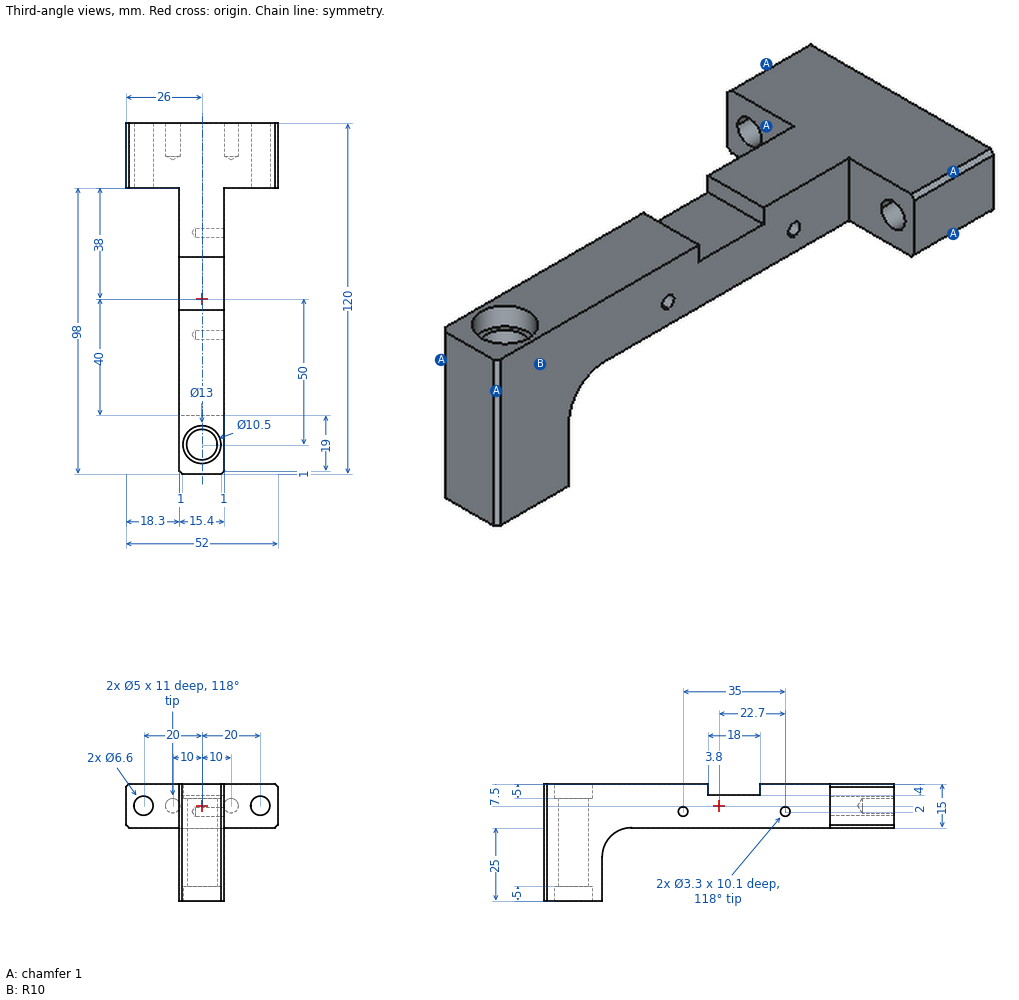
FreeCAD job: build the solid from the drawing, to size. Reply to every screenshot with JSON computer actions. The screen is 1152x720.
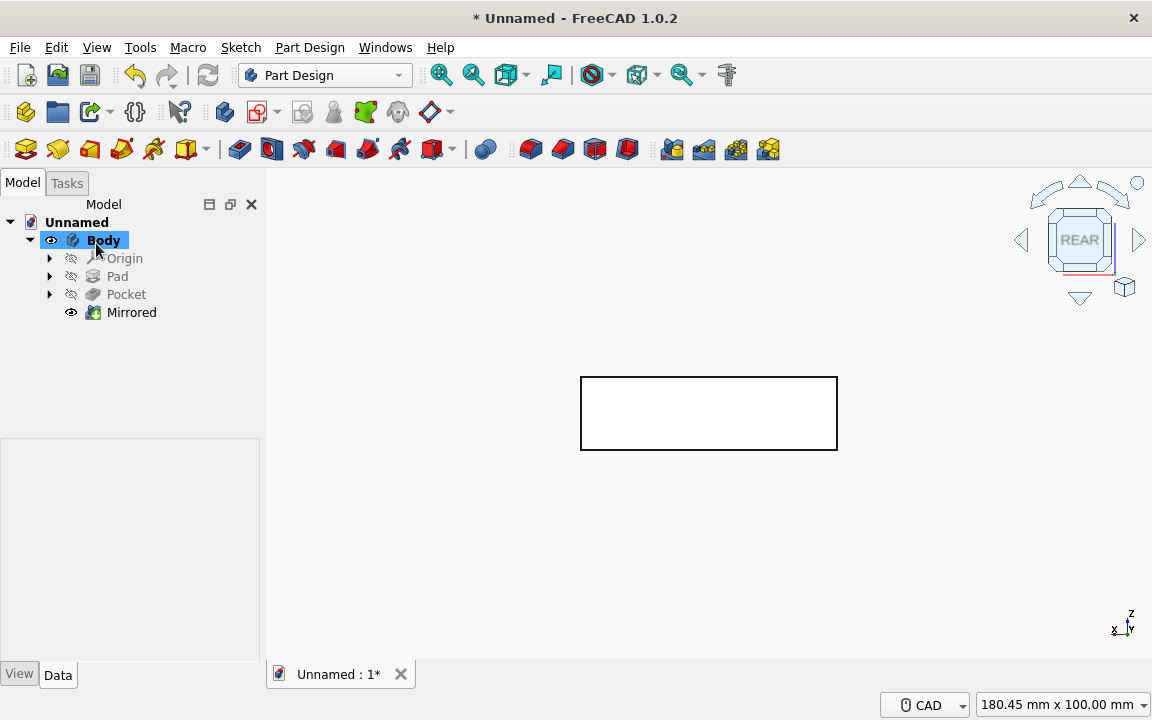
{"action": "left_click", "coordinate": [442, 76]}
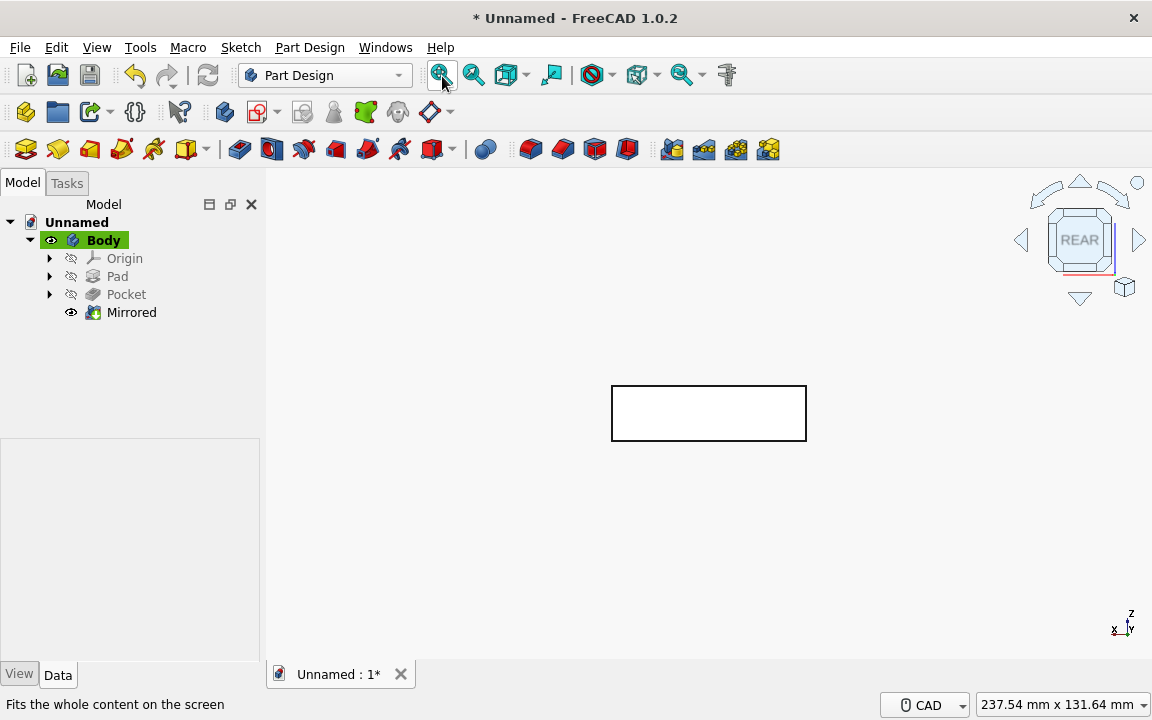
{"action": "left_click", "coordinate": [654, 413]}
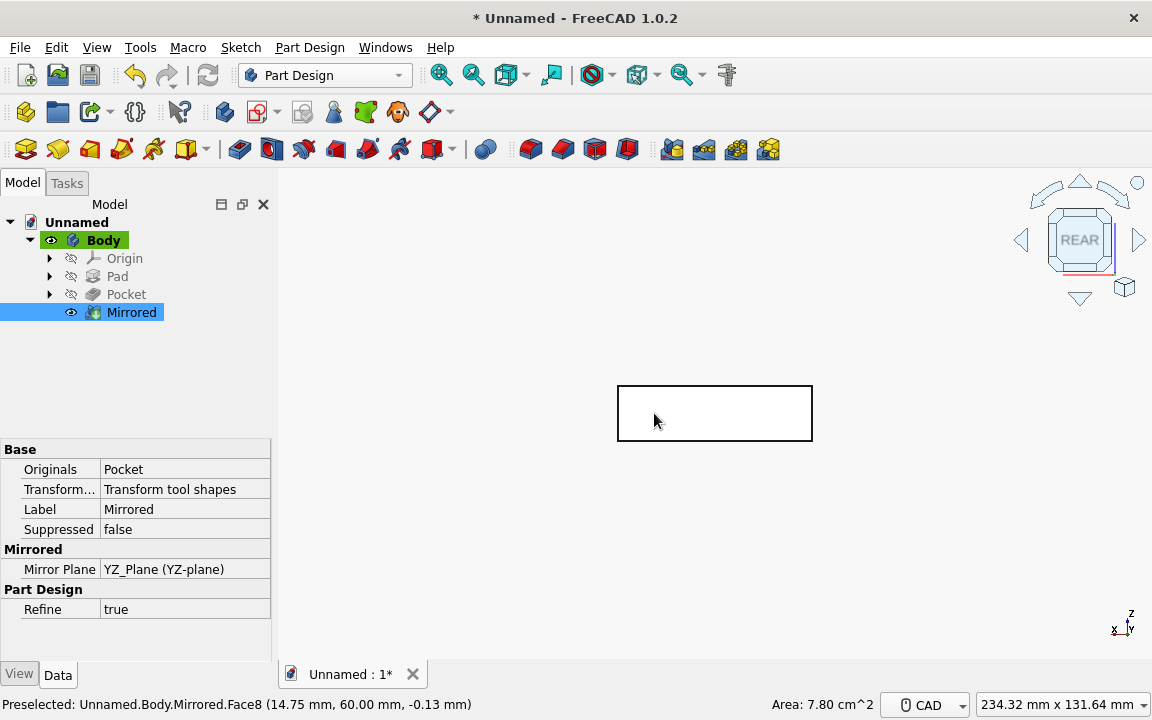
{"action": "left_click", "coordinate": [258, 112]}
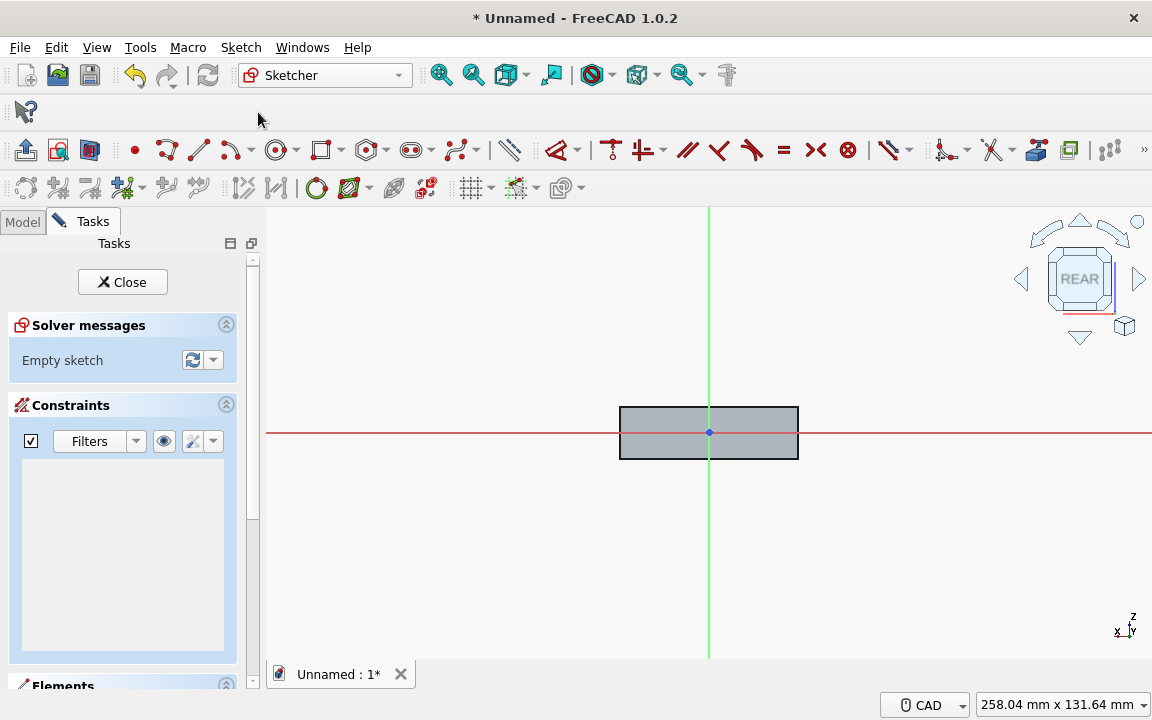
{"action": "scroll", "coordinate": [739, 433], "scroll_direction": "up", "scroll_amount": 6}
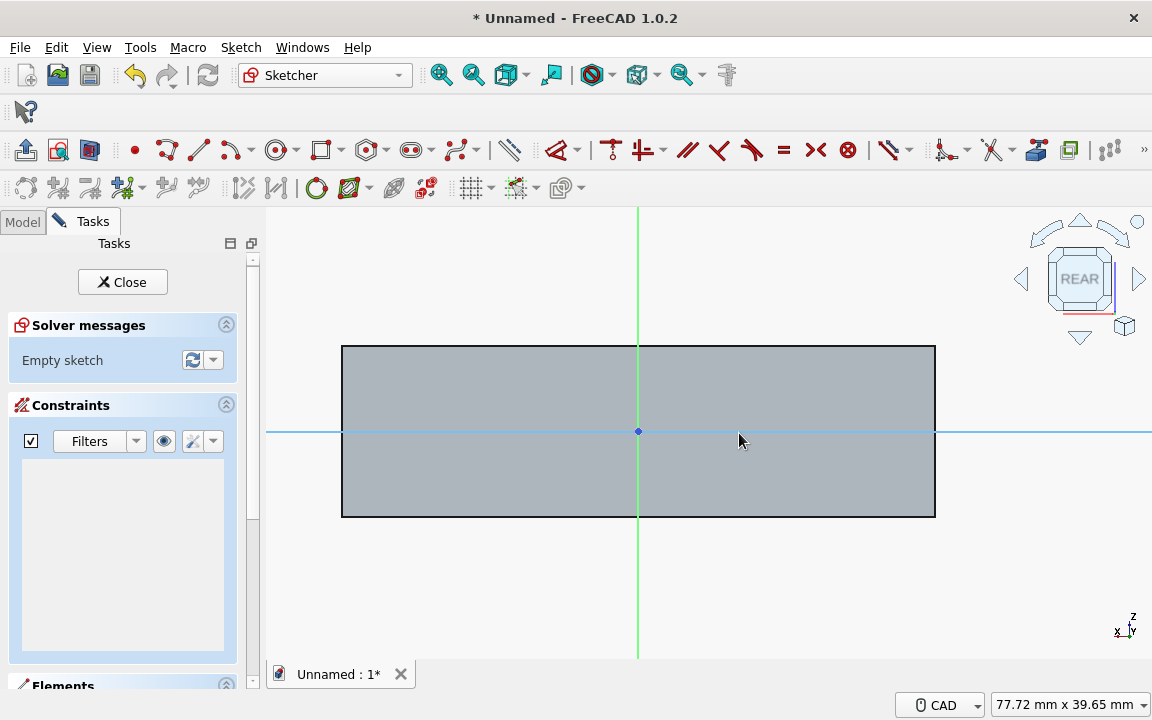
{"action": "left_click", "coordinate": [276, 150]}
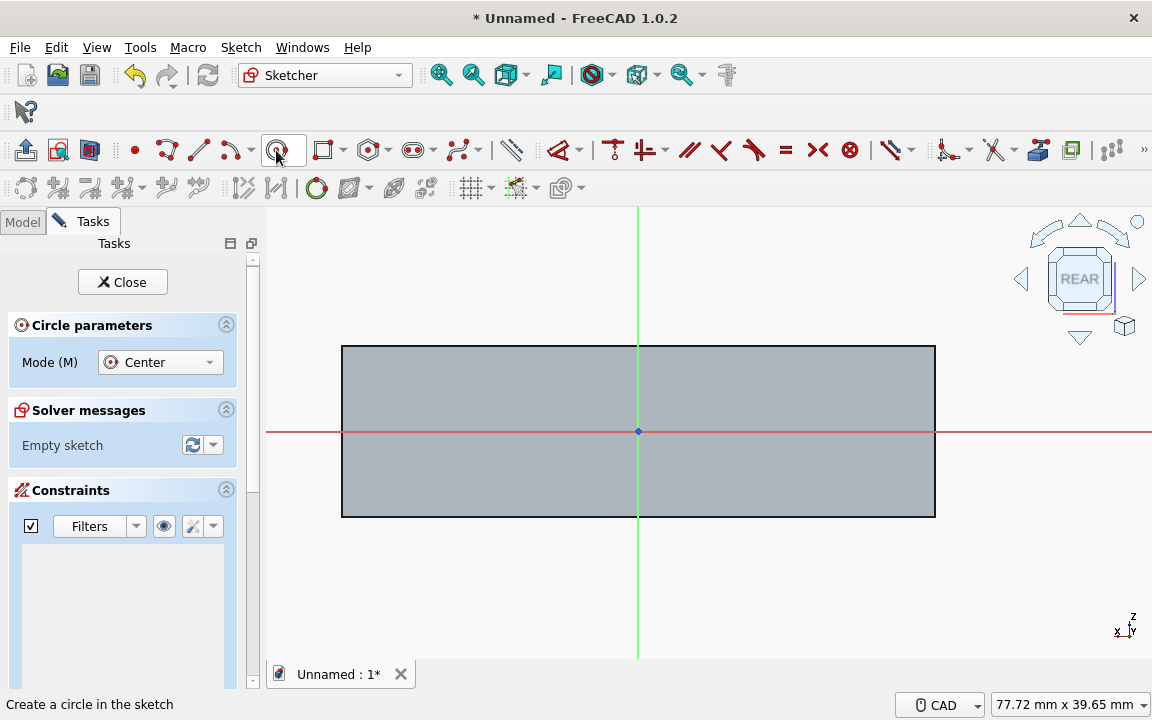
{"action": "left_click", "coordinate": [866, 432]}
{"action": "mouse_move", "coordinate": [893, 405]}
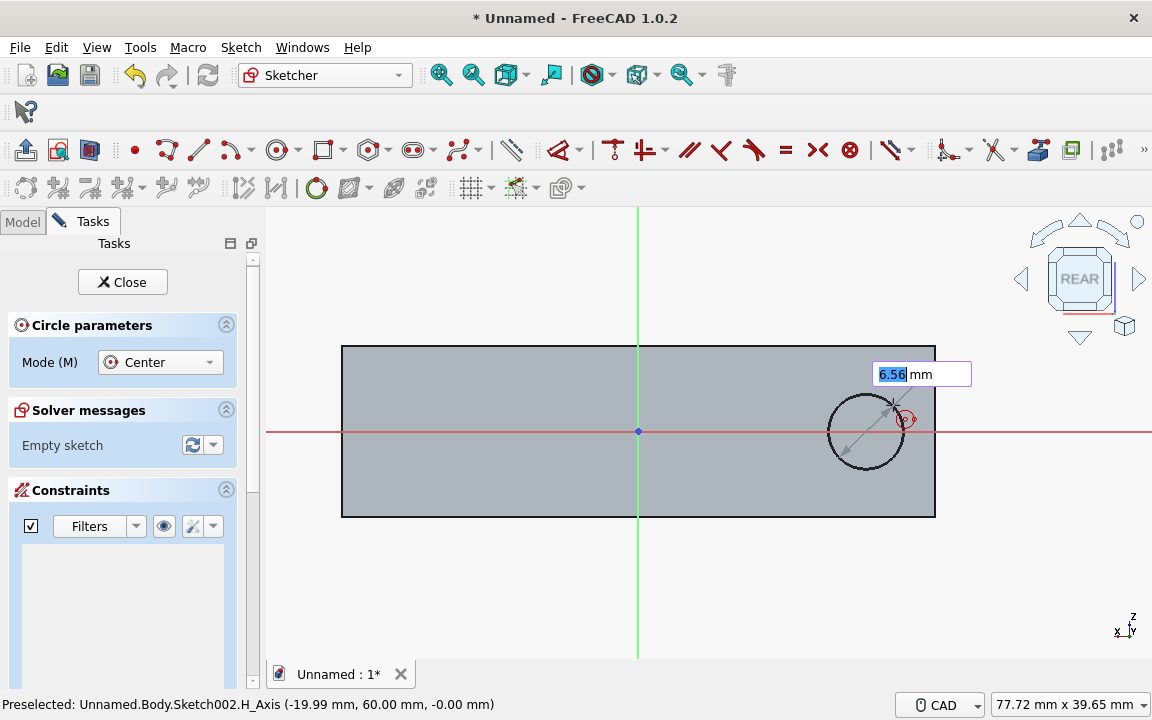
{"action": "type", "text": "6.6"}
{"action": "key", "text": "Return"}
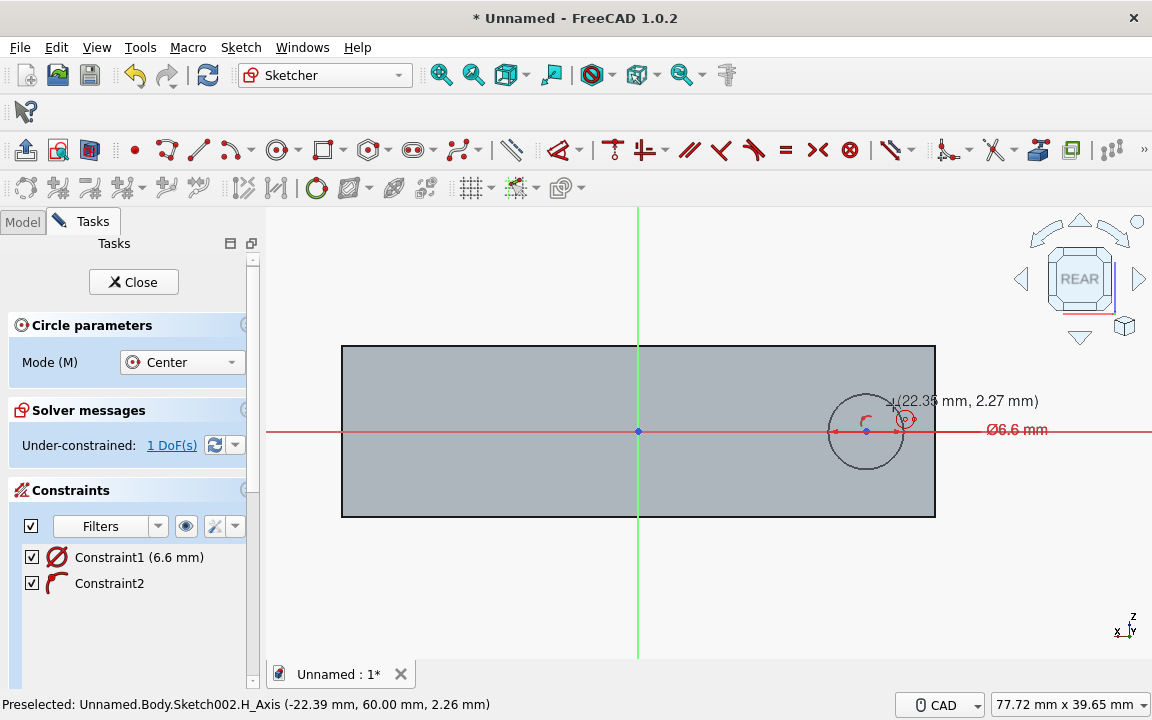
{"action": "left_click", "coordinate": [410, 432]}
{"action": "mouse_move", "coordinate": [437, 405]}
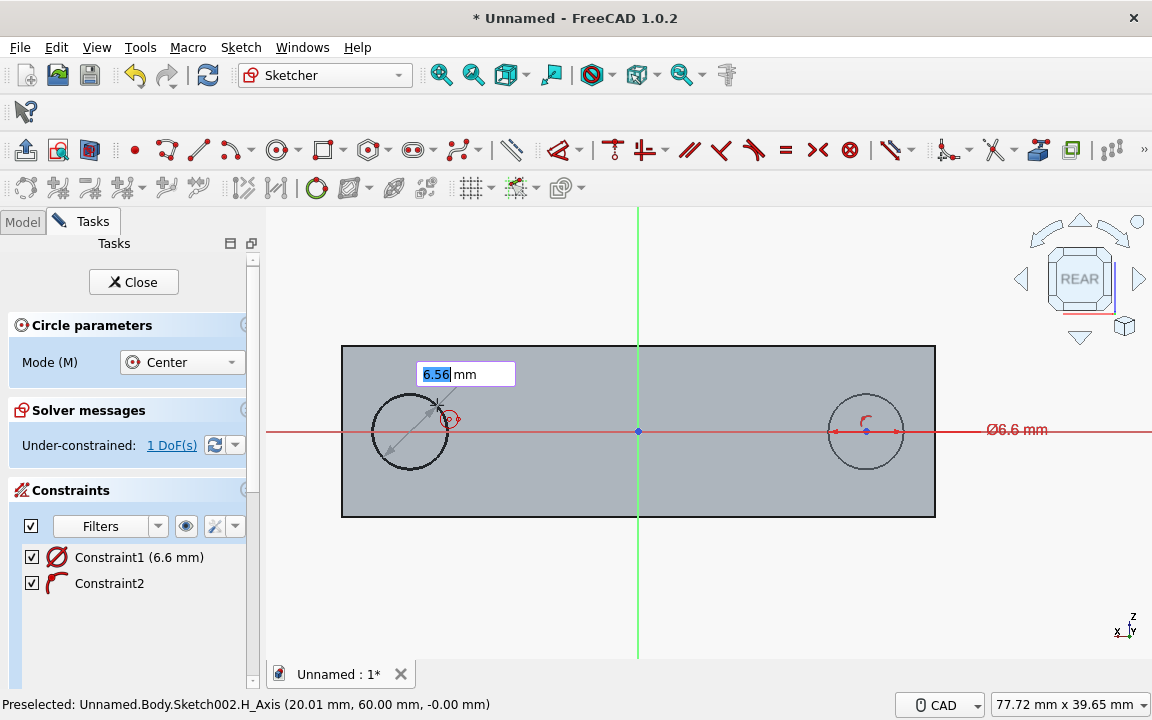
{"action": "type", "text": "6.6"}
{"action": "key", "text": "Return"}
{"action": "key", "text": "Escape"}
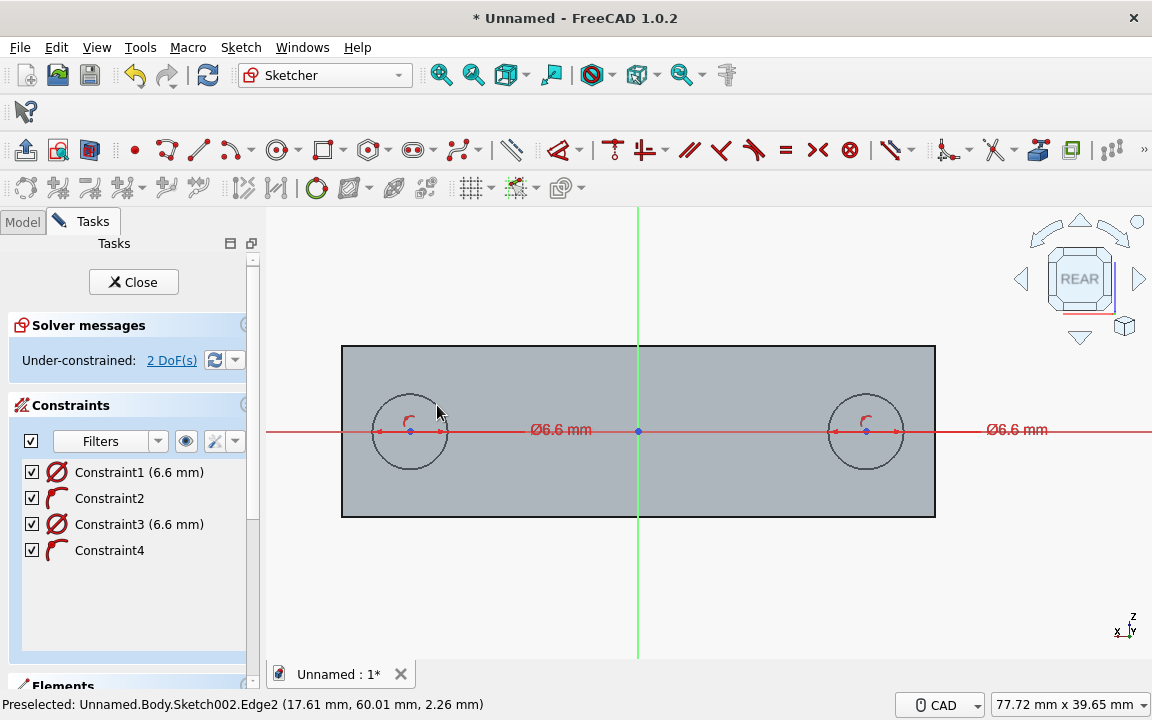
{"action": "left_click", "coordinate": [558, 150]}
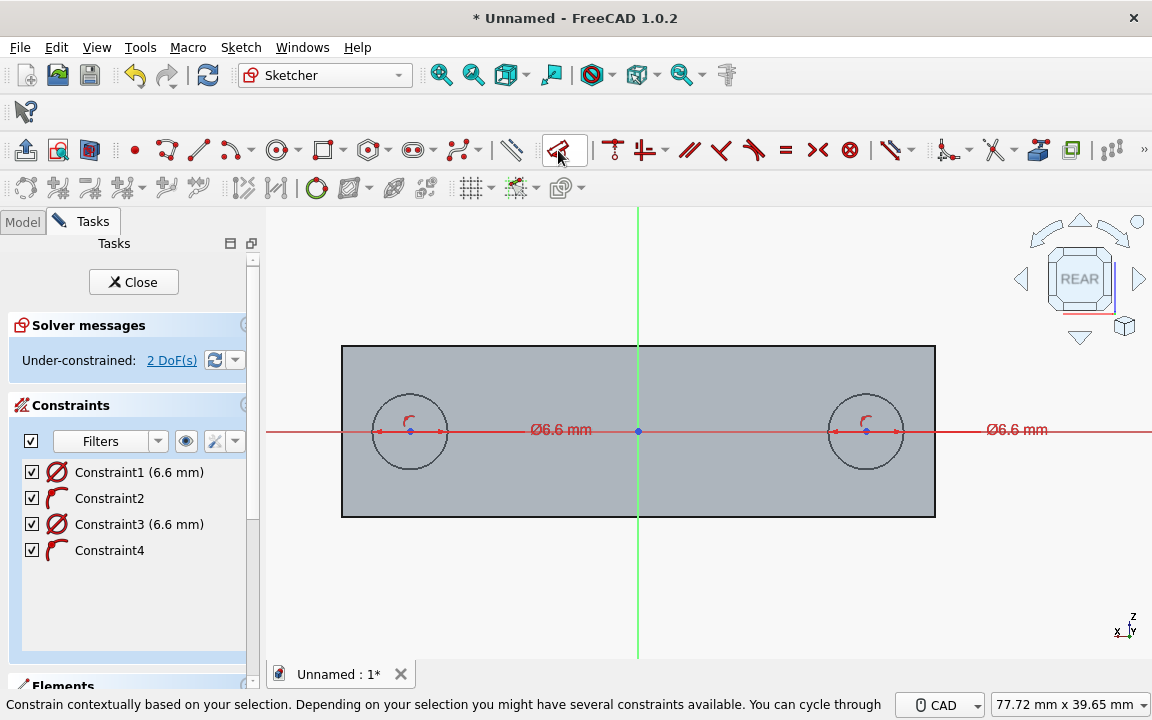
{"action": "left_click", "coordinate": [866, 432]}
{"action": "left_click", "coordinate": [752, 466]}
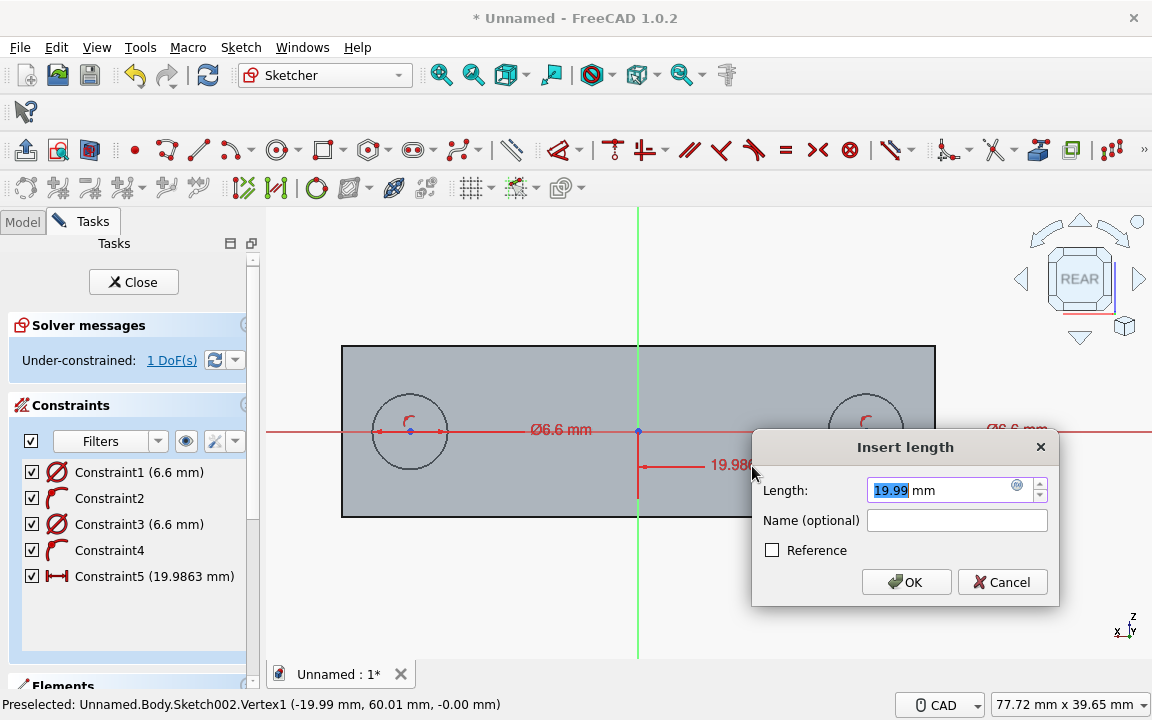
{"action": "type", "text": "20"}
{"action": "key", "text": "Return"}